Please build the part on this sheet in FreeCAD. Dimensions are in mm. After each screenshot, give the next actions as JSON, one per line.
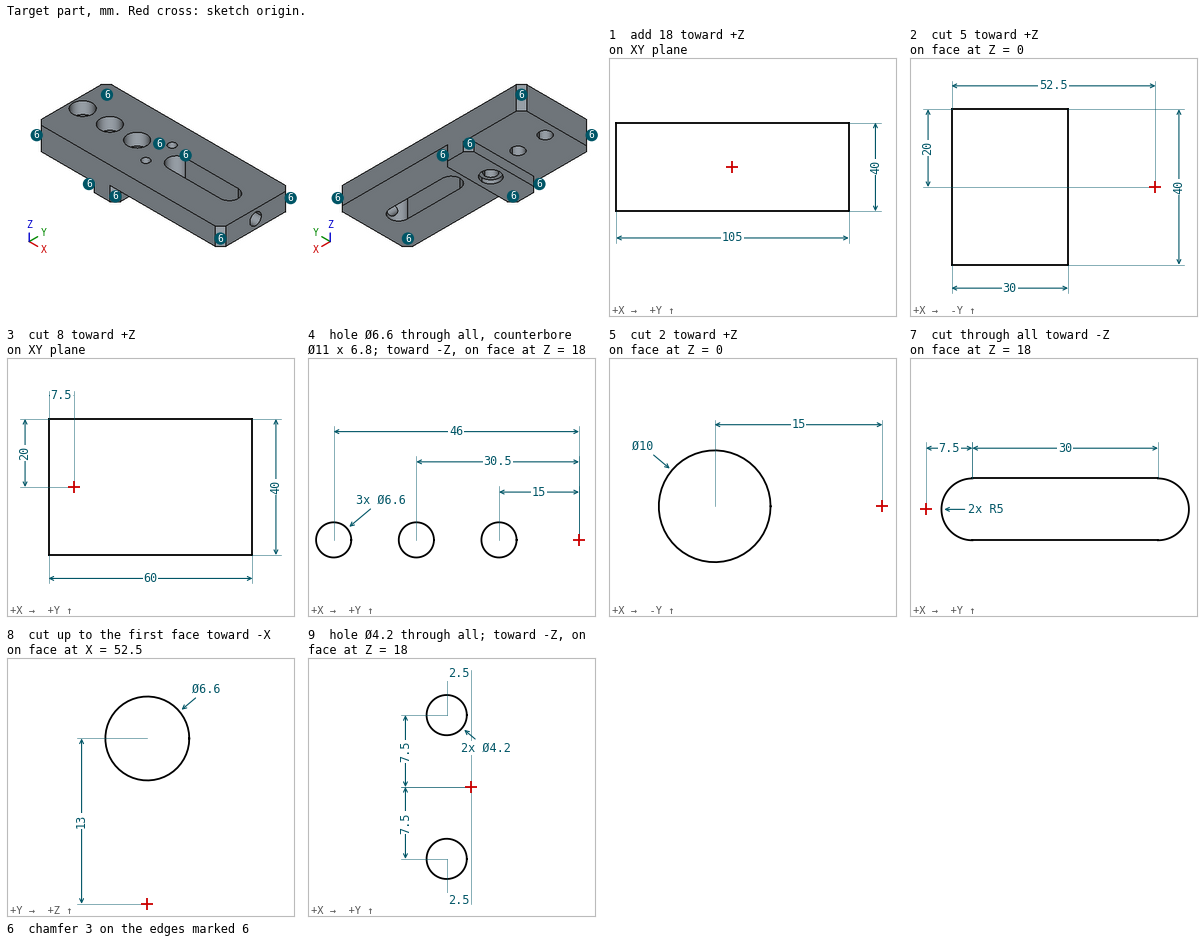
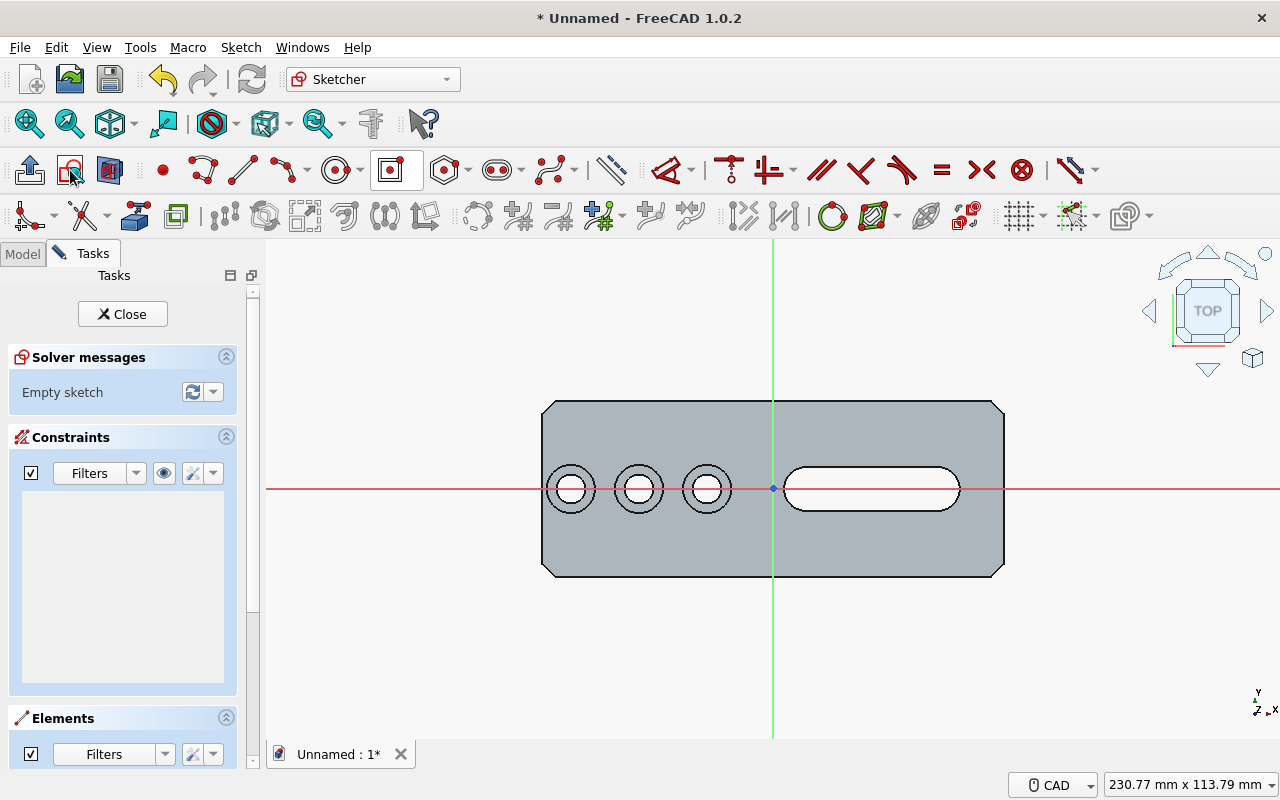
{"action": "scroll", "coordinate": [782, 489], "scroll_direction": "up", "scroll_amount": 7}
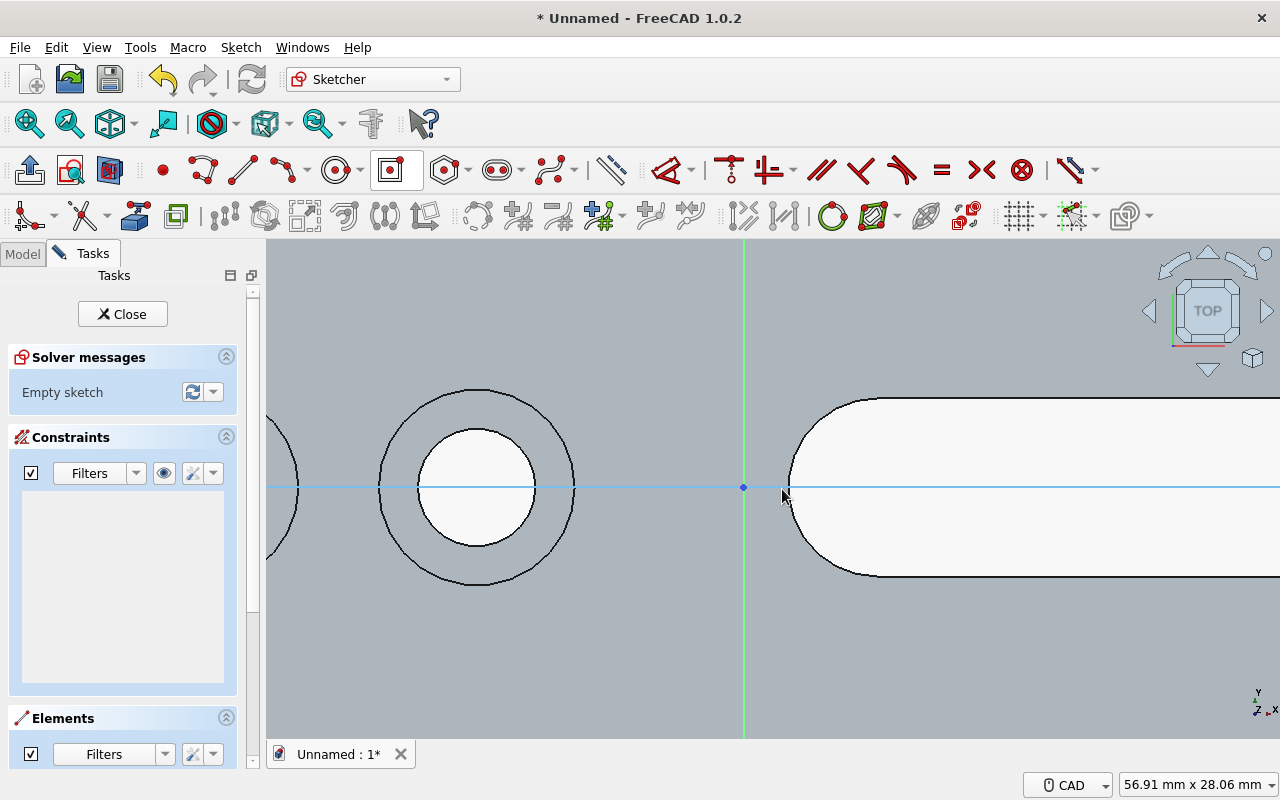
{"action": "key", "text": "g c"}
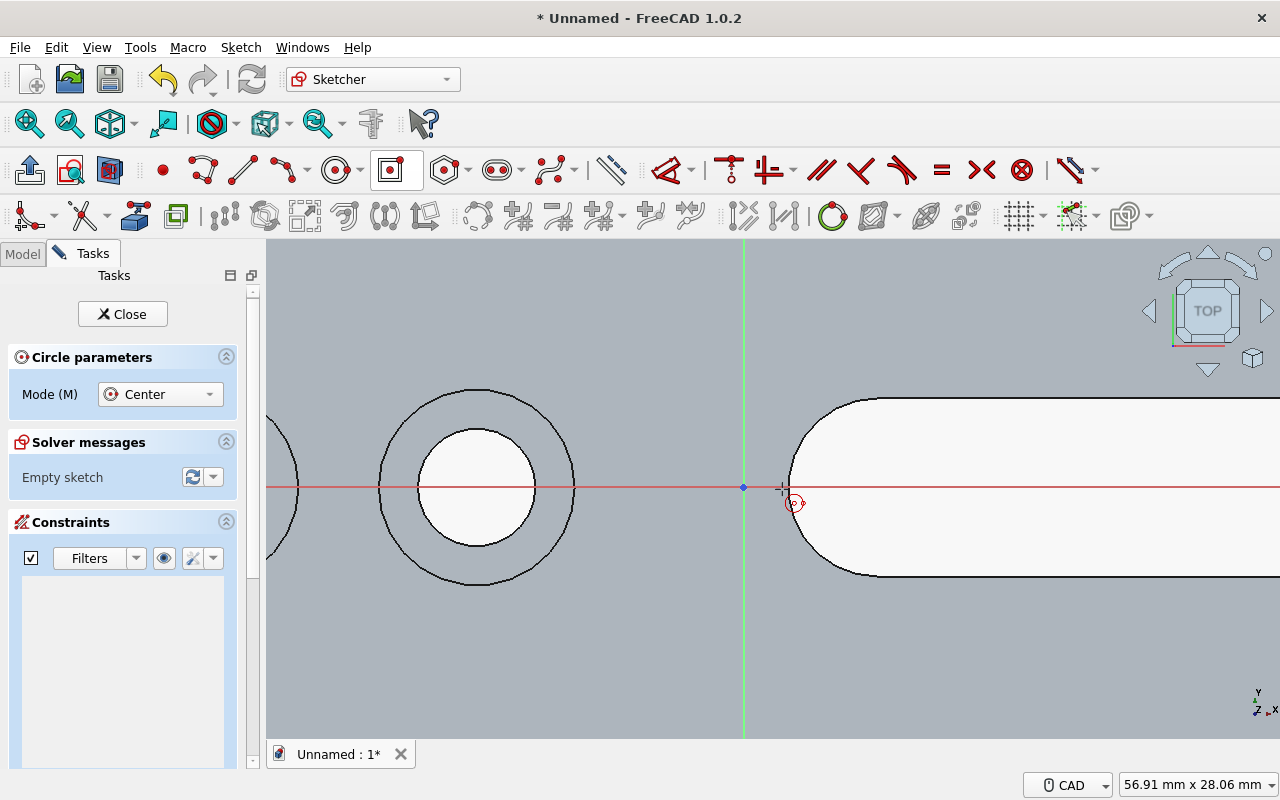
{"action": "left_click", "coordinate": [699, 354]}
{"action": "mouse_move", "coordinate": [726, 327]}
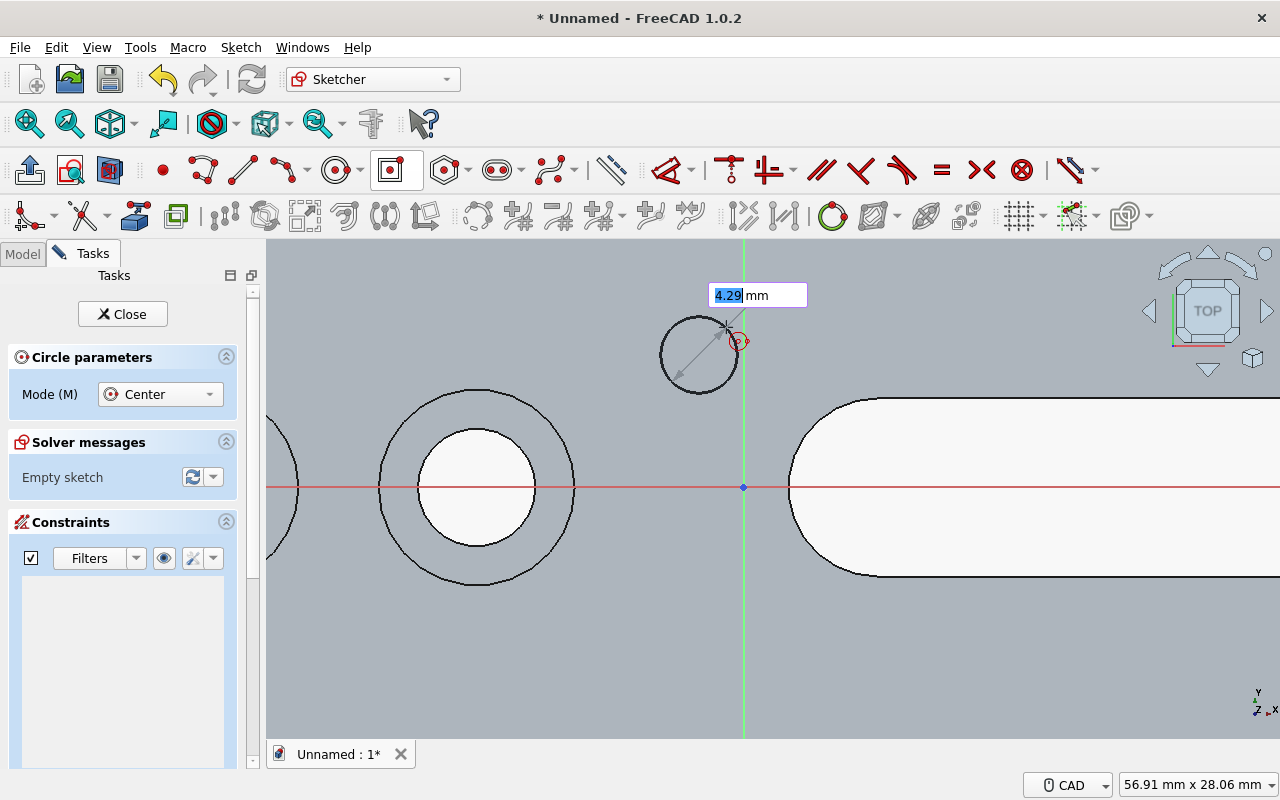
{"action": "type", "text": "4.2"}
{"action": "key", "text": "Return"}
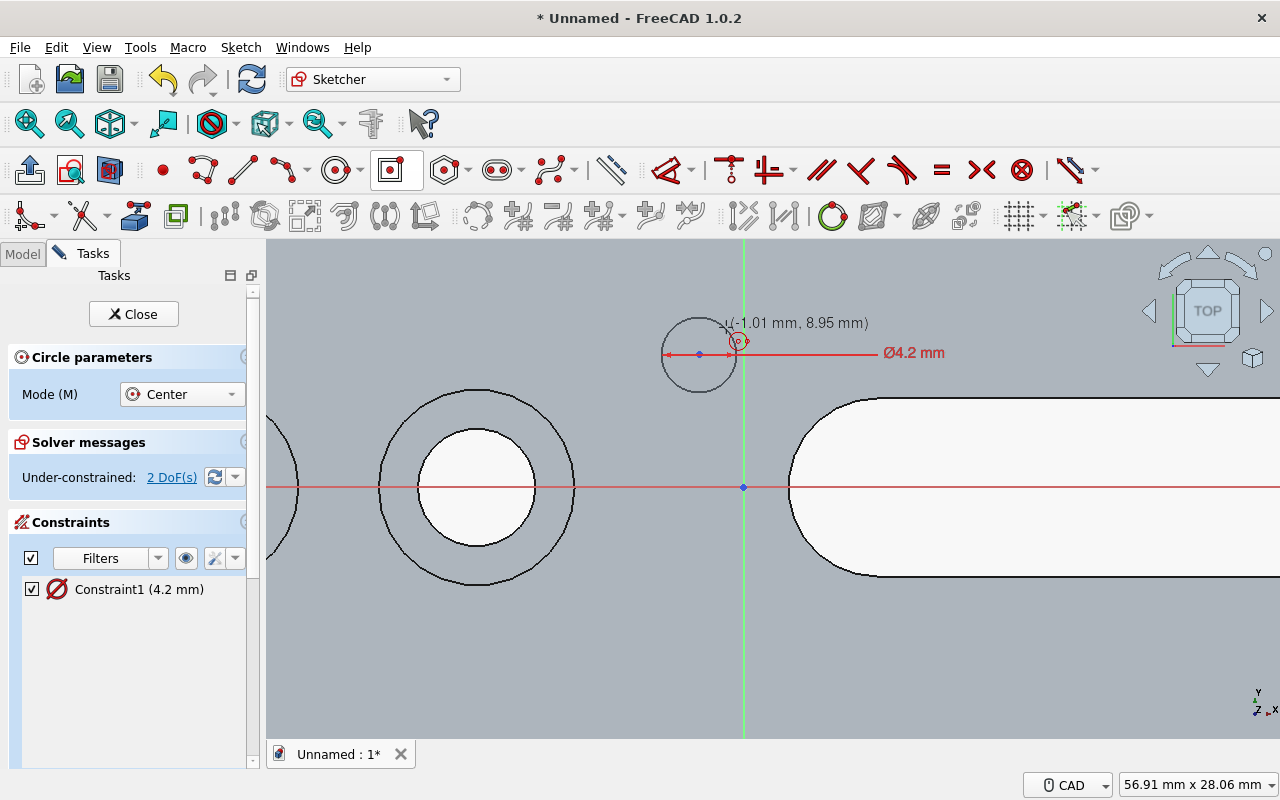
{"action": "left_click", "coordinate": [699, 621]}
{"action": "mouse_move", "coordinate": [726, 595]}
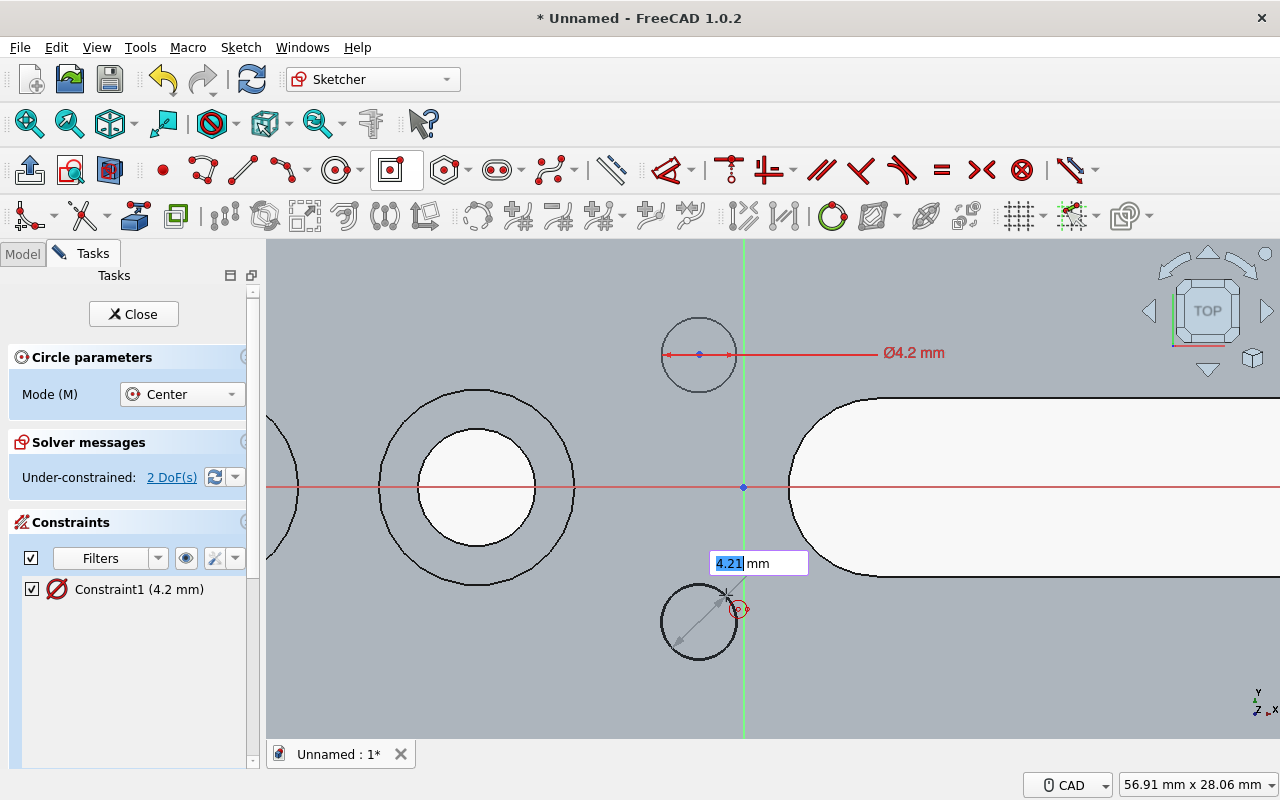
{"action": "type", "text": "4.2"}
{"action": "key", "text": "Return"}
{"action": "key", "text": "Escape"}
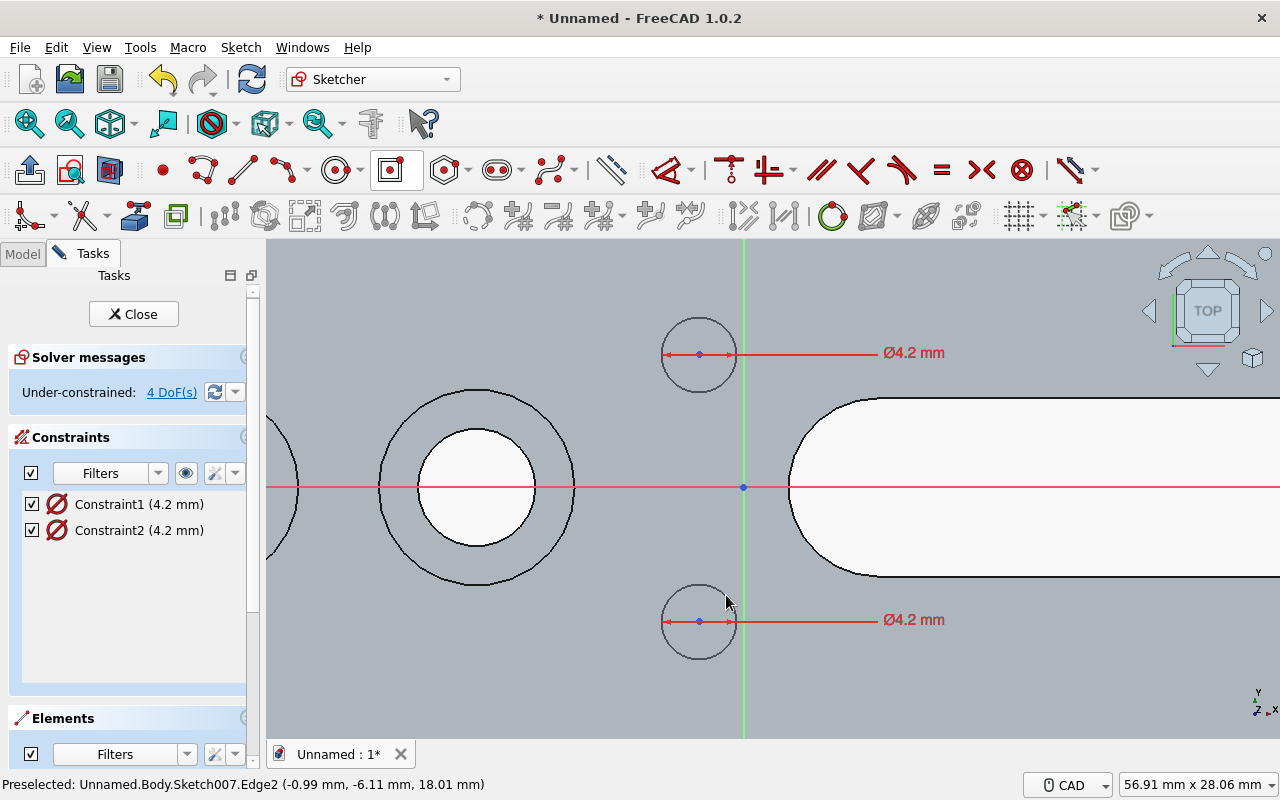
{"action": "left_click", "coordinate": [666, 170]}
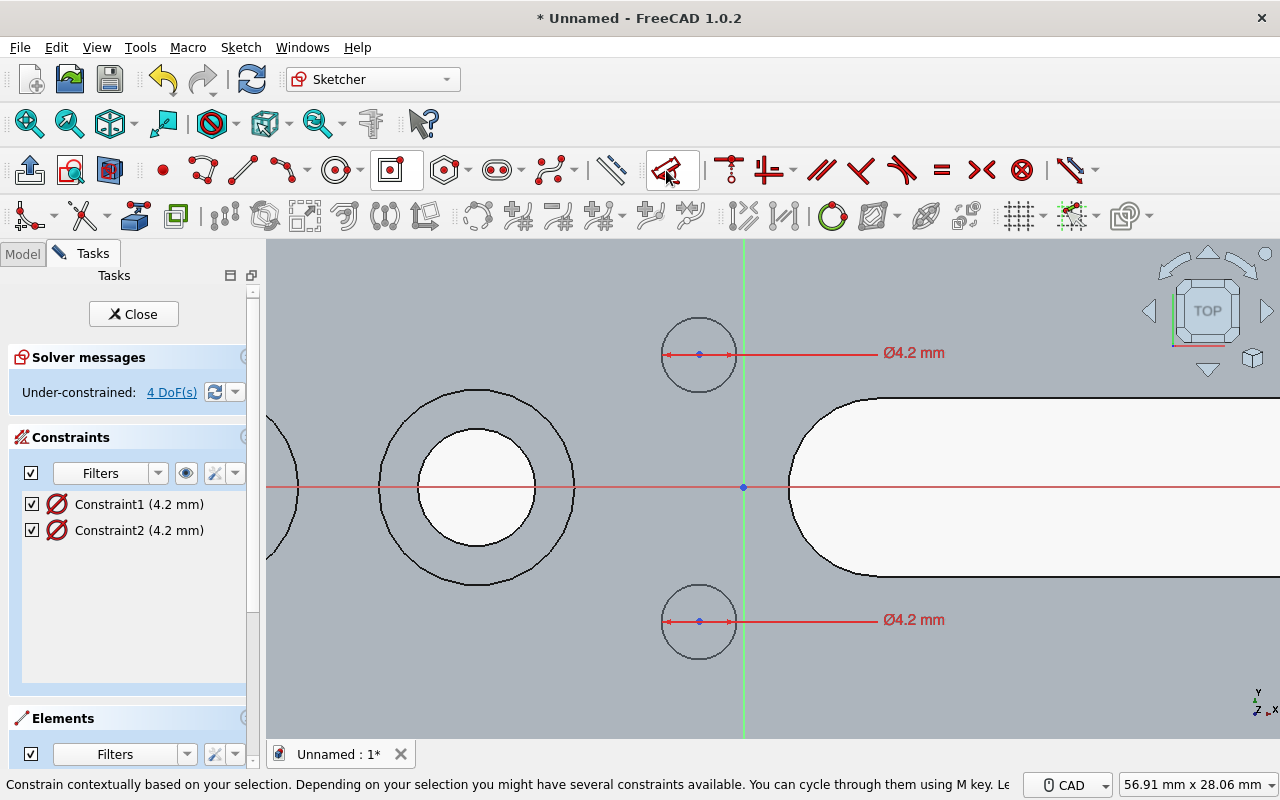
{"action": "left_click", "coordinate": [699, 355]}
{"action": "left_click", "coordinate": [721, 521]}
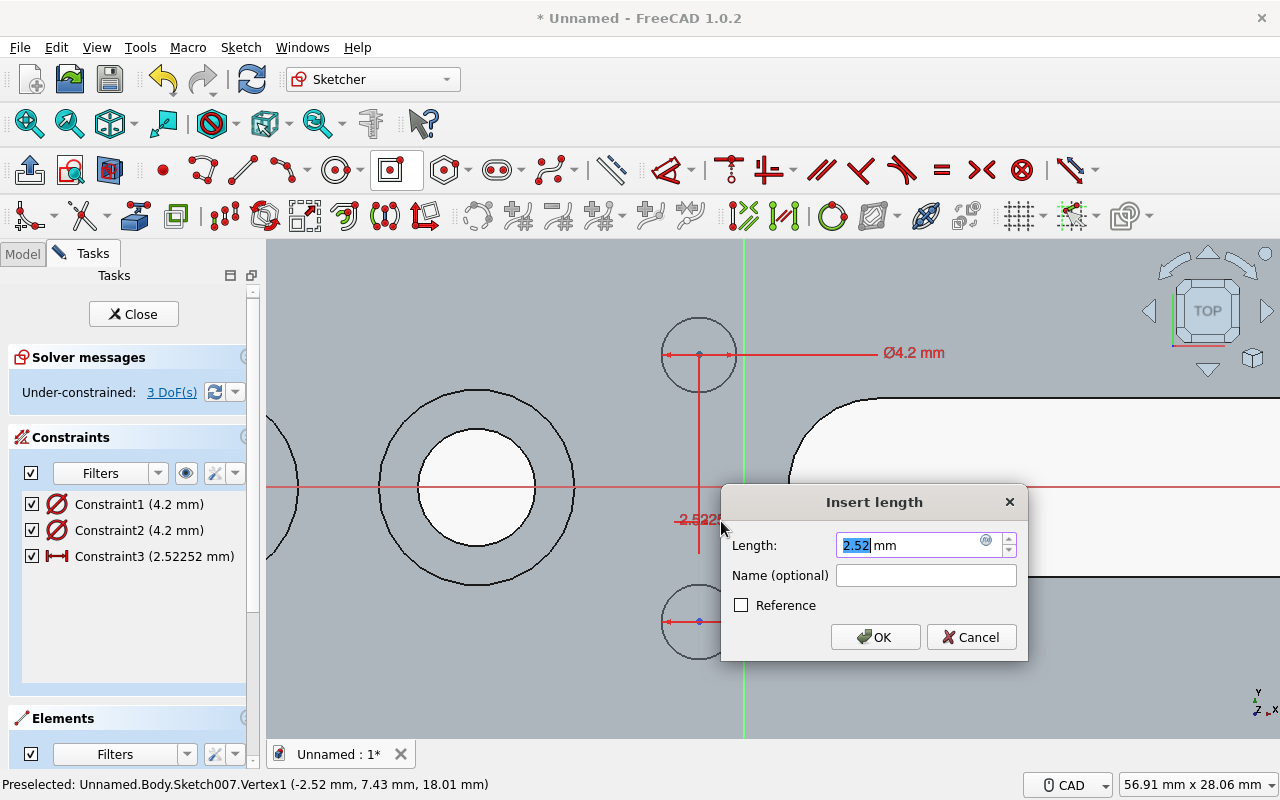
{"action": "type", "text": "2.5"}
{"action": "key", "text": "Return"}